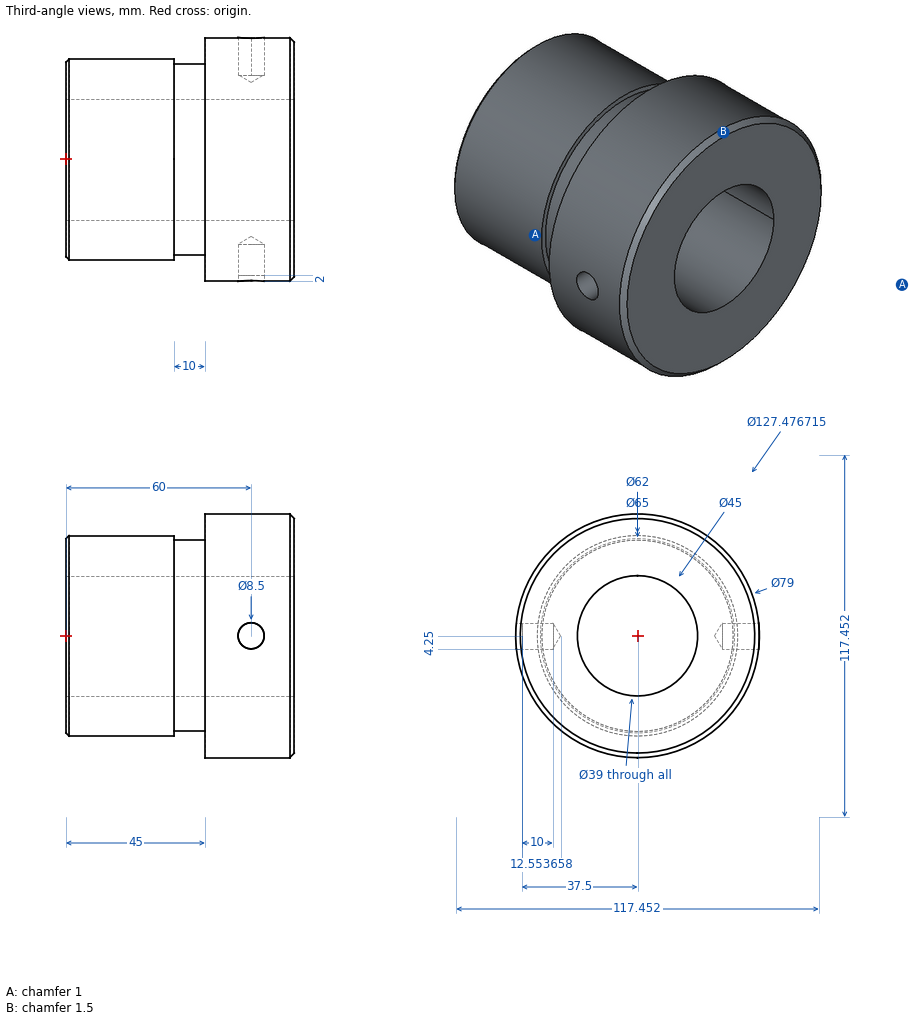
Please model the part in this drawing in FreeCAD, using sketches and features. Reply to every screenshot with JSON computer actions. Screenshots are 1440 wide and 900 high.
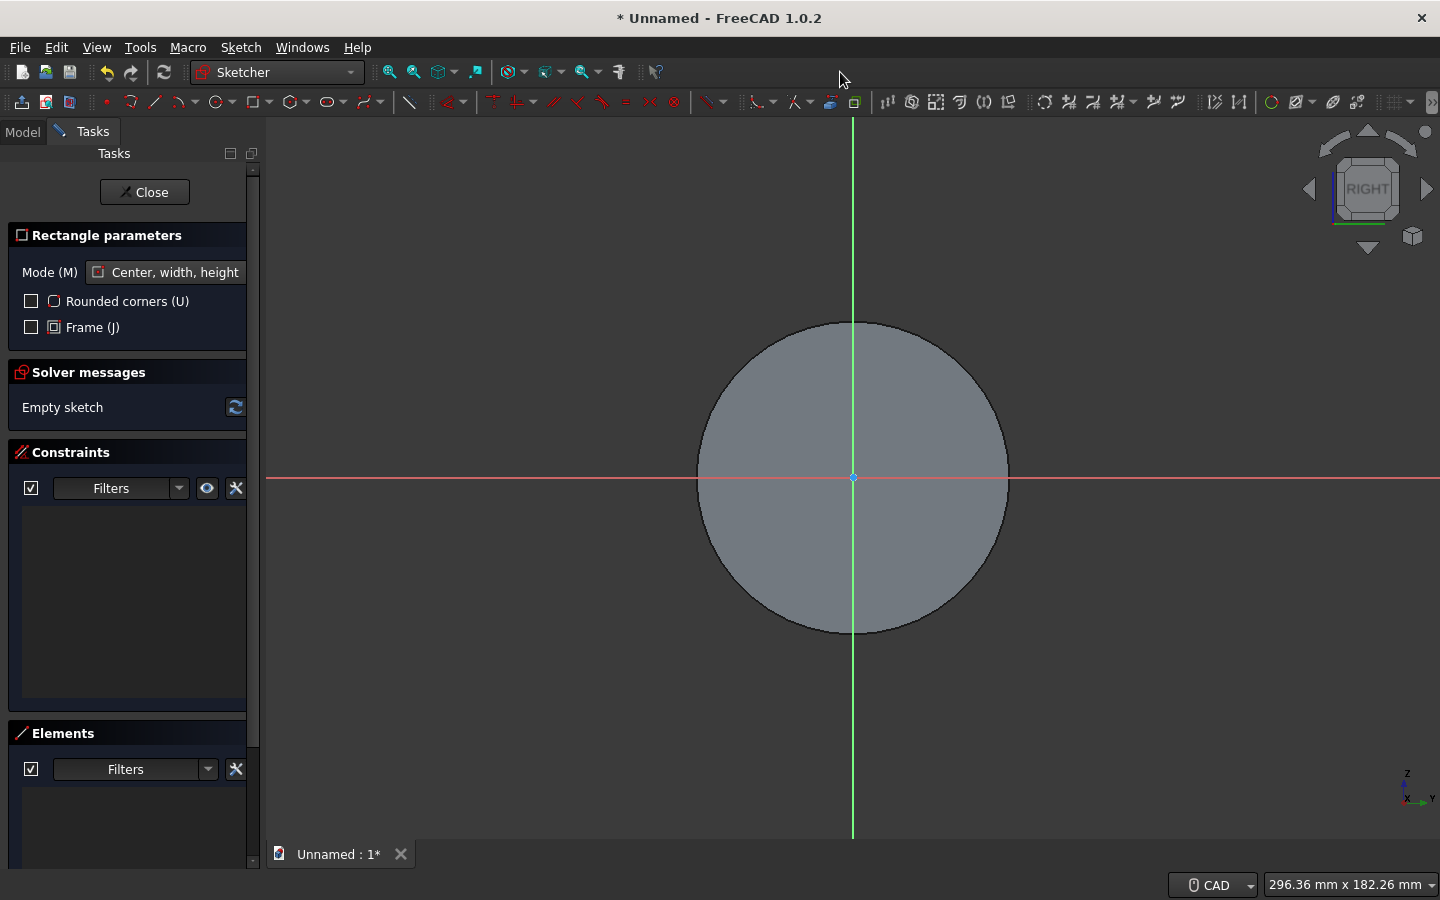
{"action": "left_click", "coordinate": [853, 478]}
{"action": "mouse_move", "coordinate": [1086, 245]}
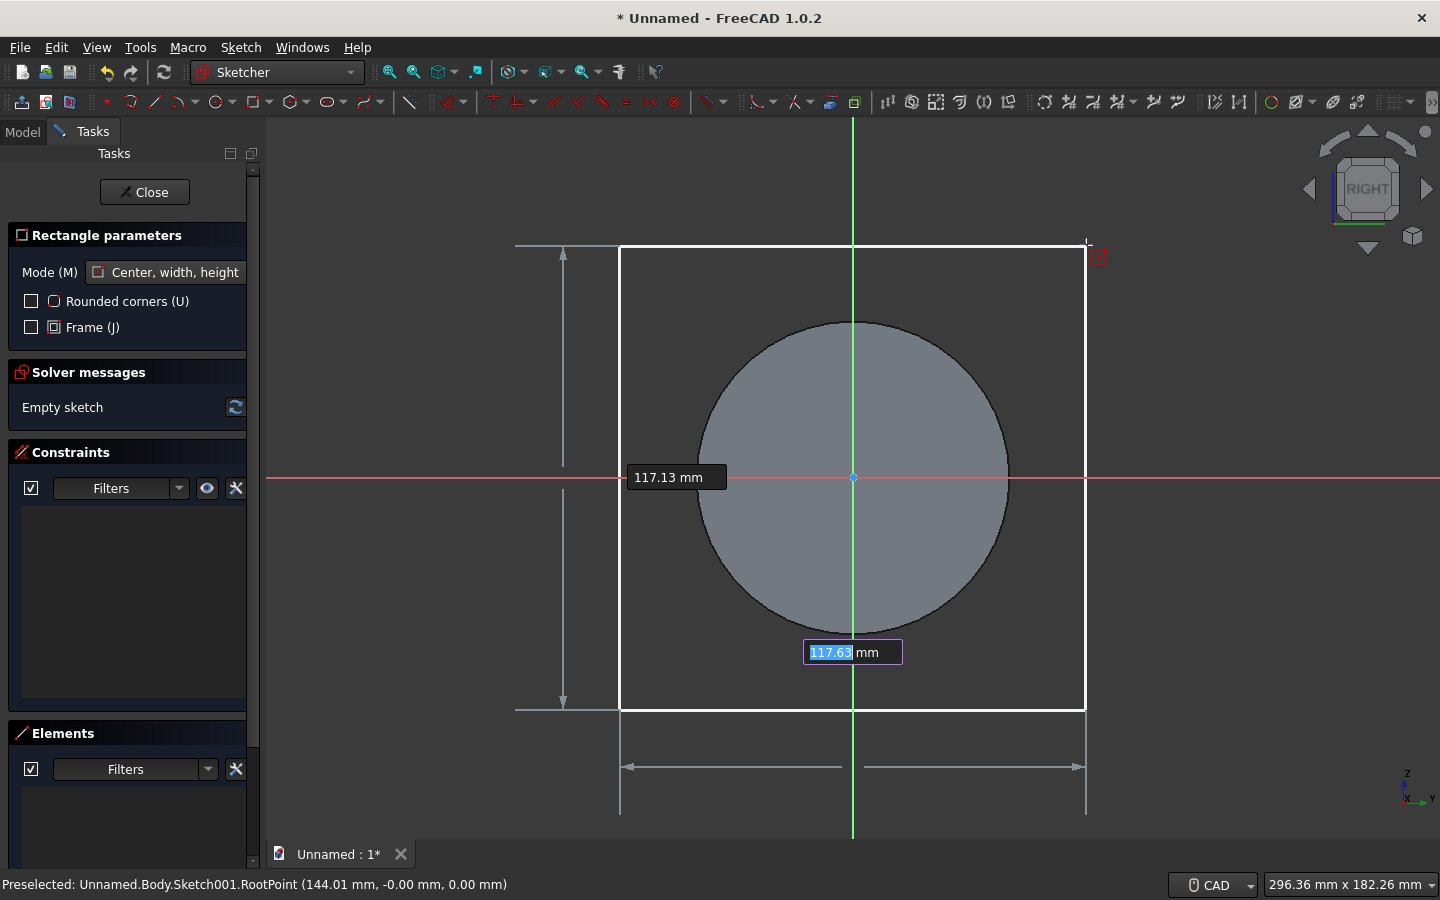
{"action": "type", "text": "117.452"}
{"action": "key", "text": "Tab"}
{"action": "type", "text": "117.452"}
{"action": "key", "text": "Return"}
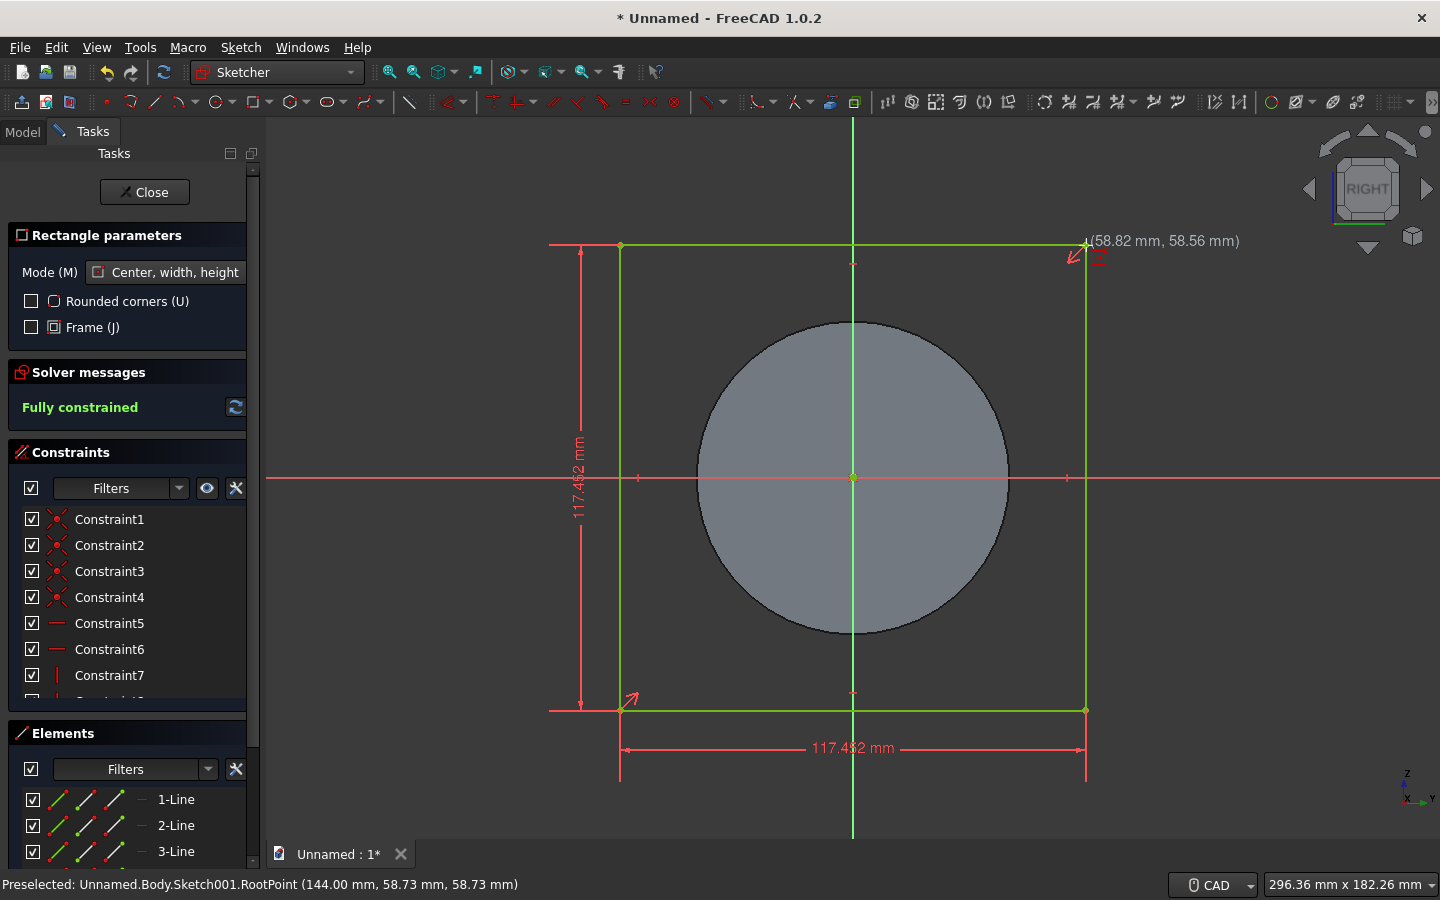
{"action": "key", "text": "g c"}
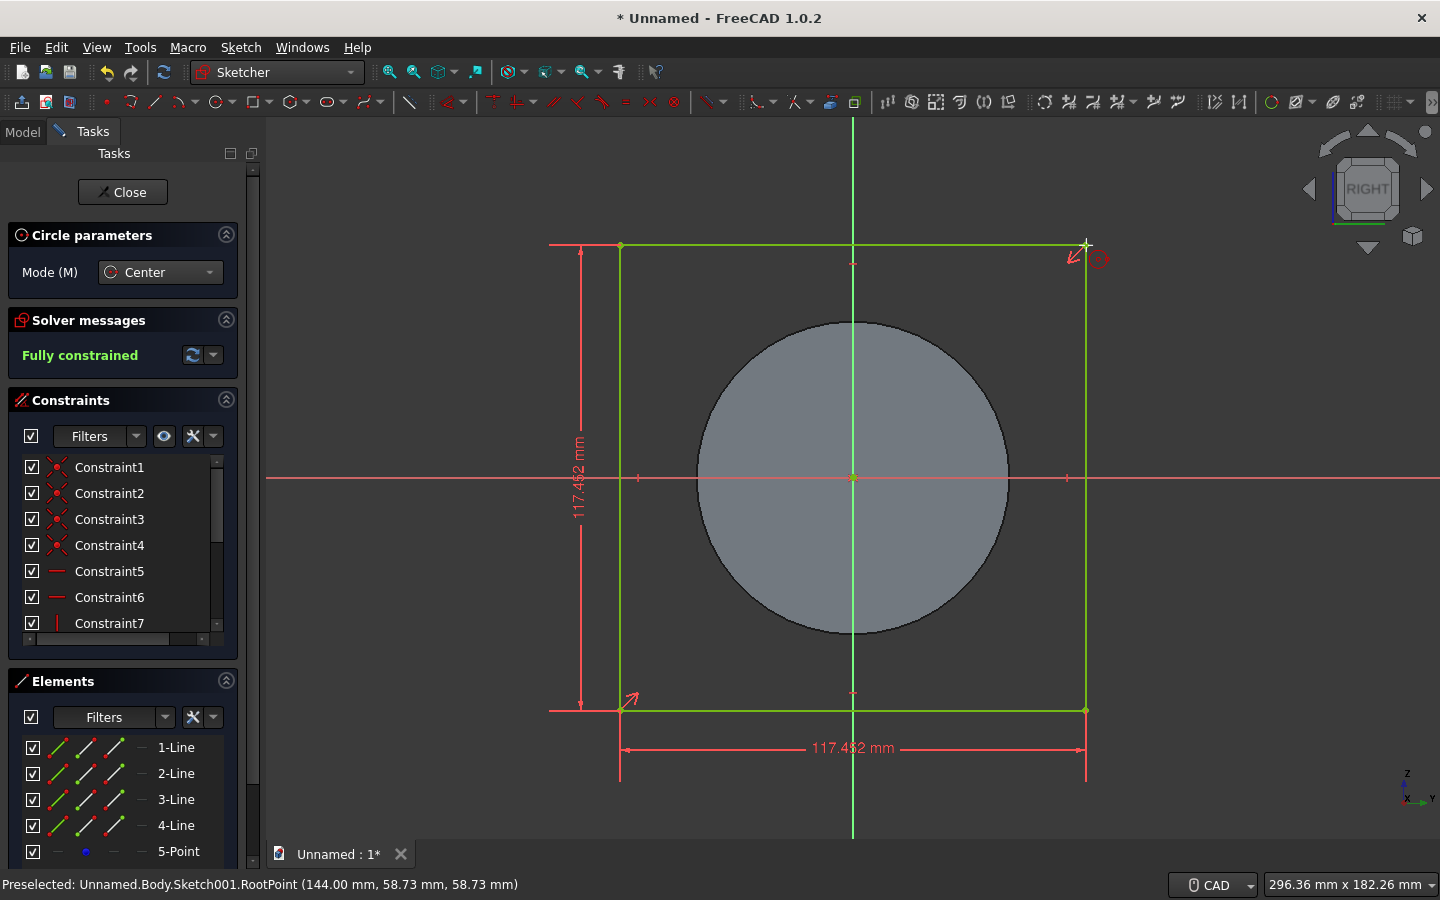
{"action": "left_click", "coordinate": [853, 478]}
{"action": "mouse_move", "coordinate": [916, 415]}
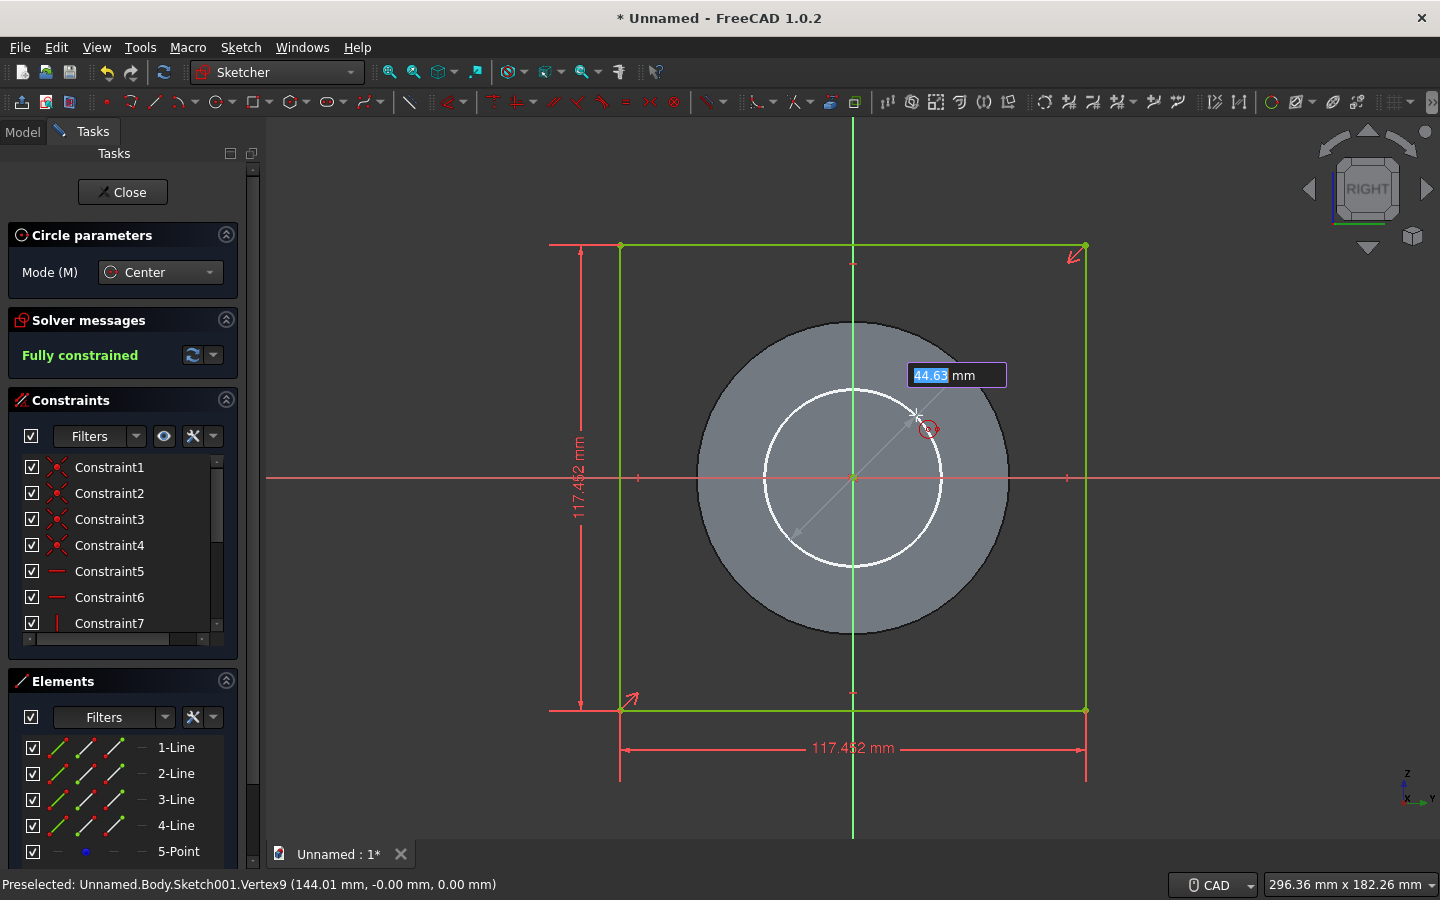
{"action": "type", "text": "45"}
{"action": "key", "text": "Return"}
{"action": "key", "text": "Escape"}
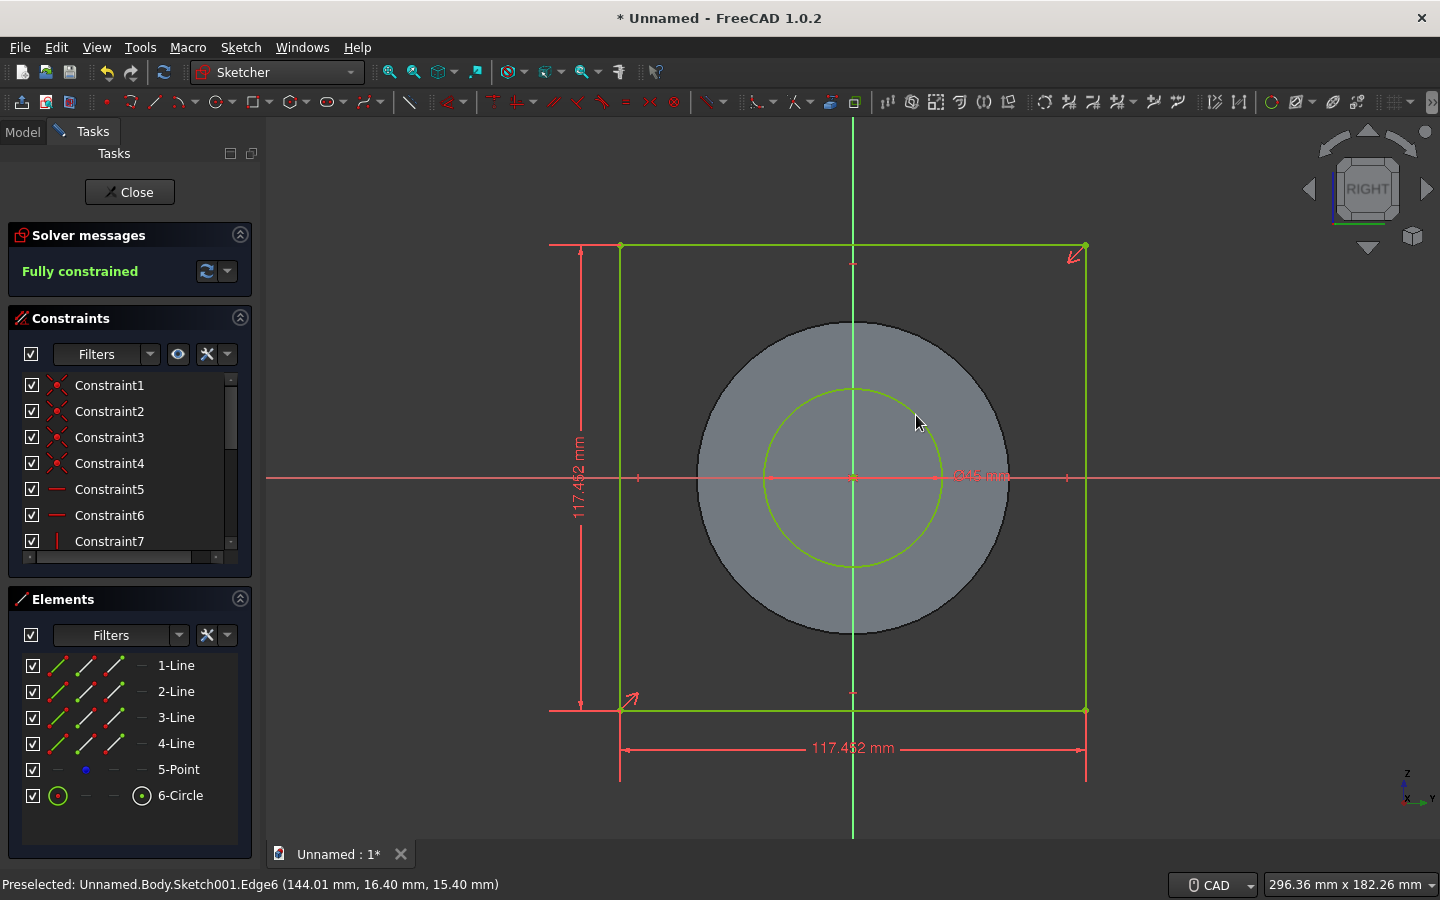
{"action": "left_click", "coordinate": [130, 192]}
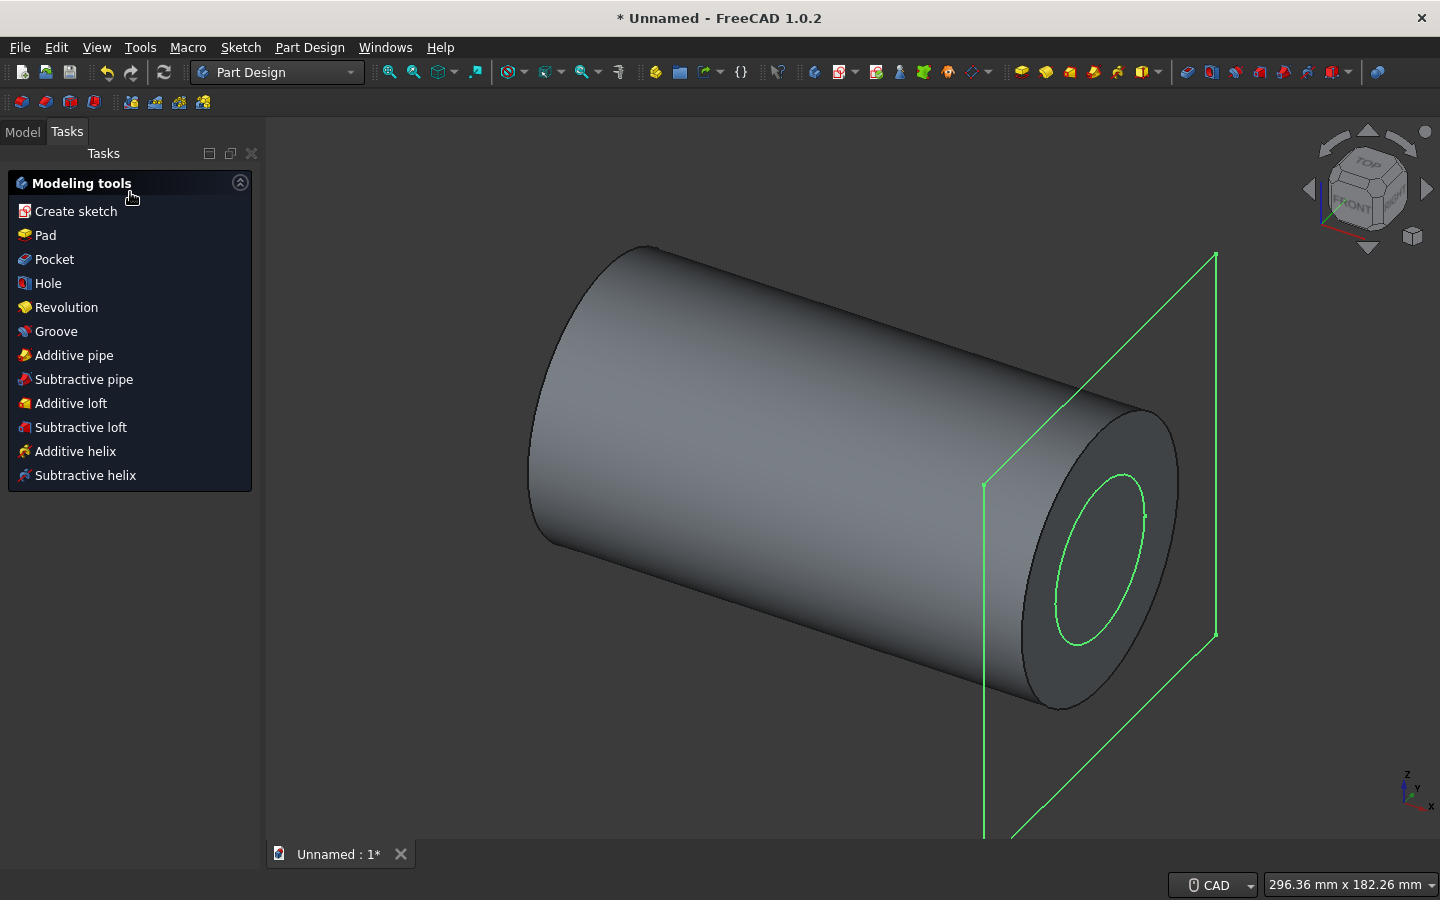
{"action": "left_click", "coordinate": [1188, 72]}